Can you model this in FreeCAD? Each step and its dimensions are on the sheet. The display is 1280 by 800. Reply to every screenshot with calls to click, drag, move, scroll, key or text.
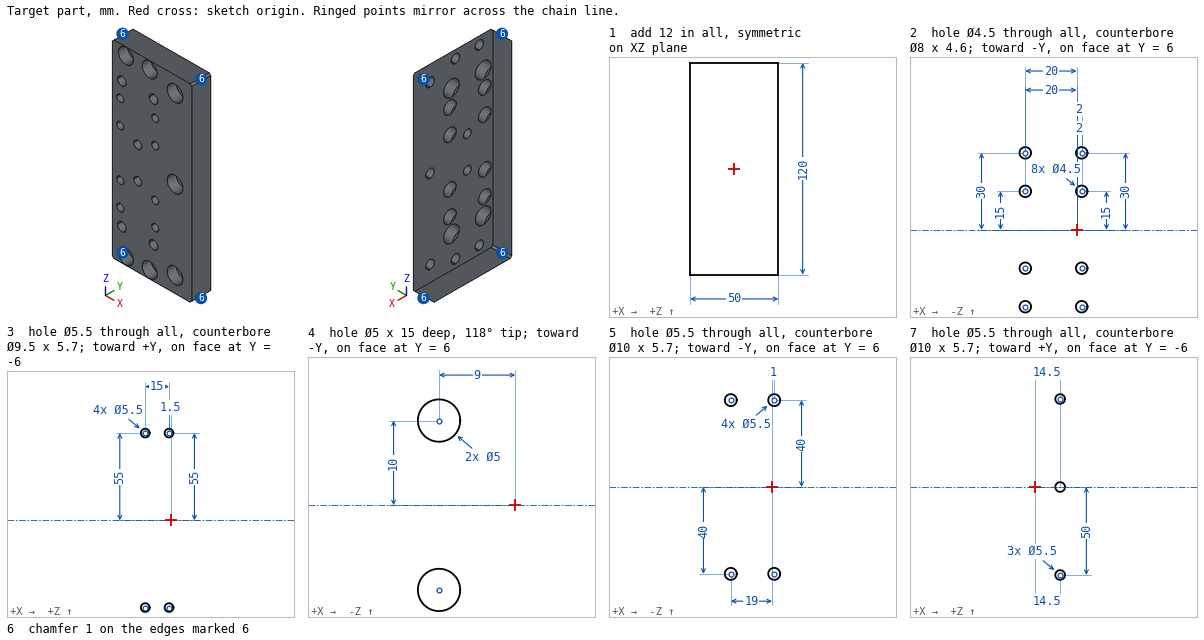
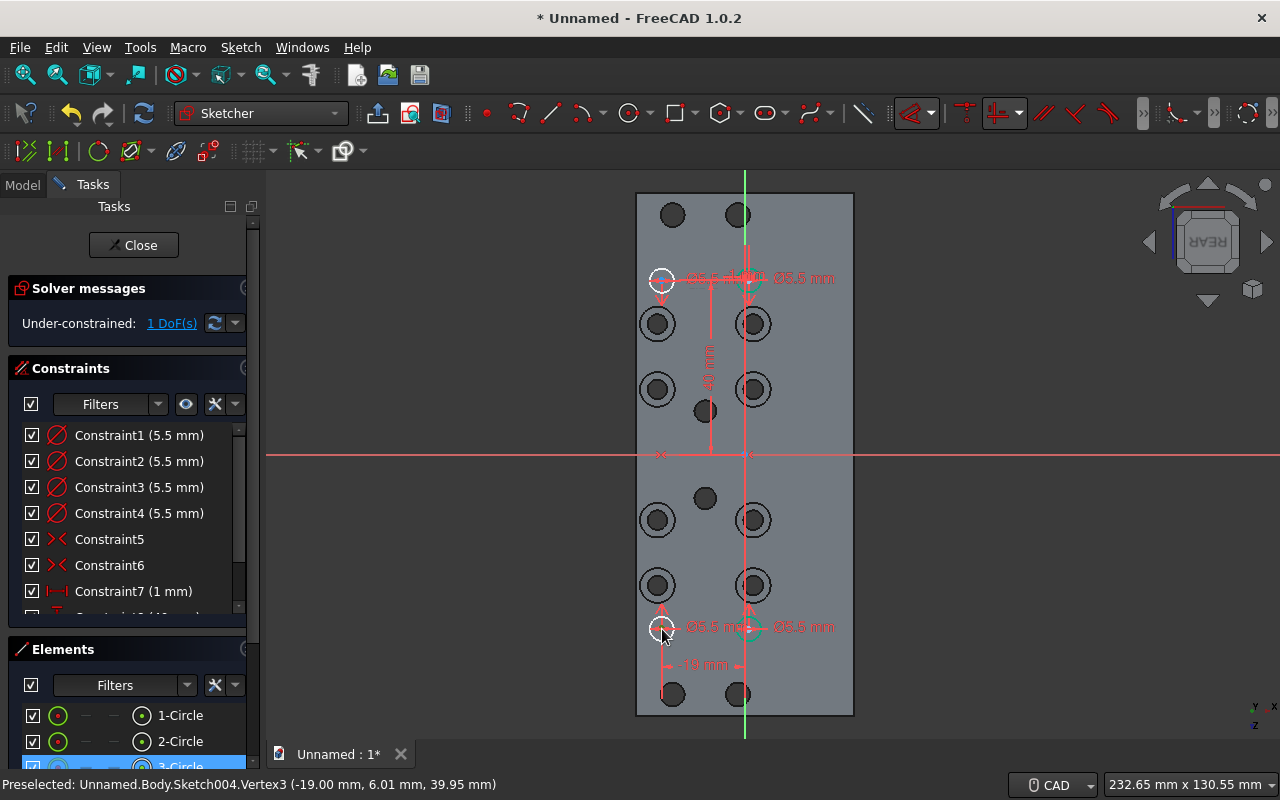
click(934, 114)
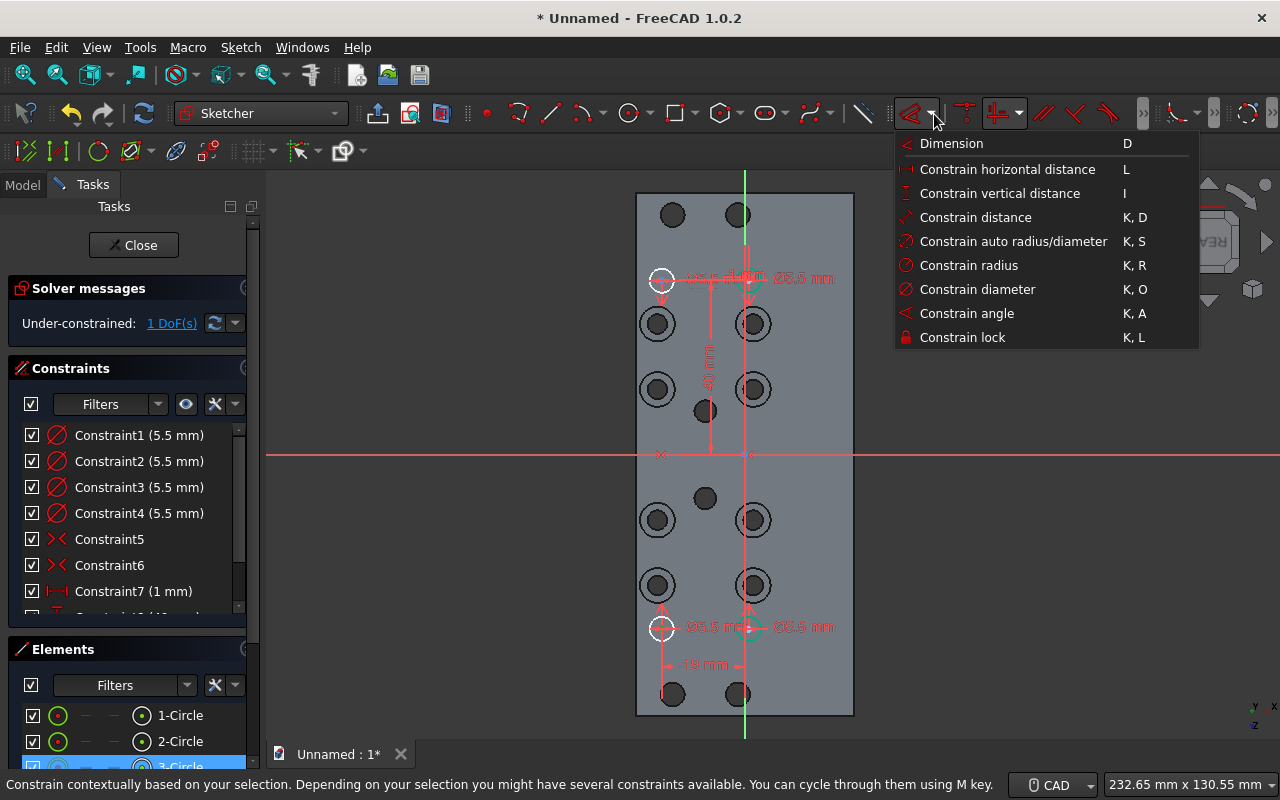
click(1047, 193)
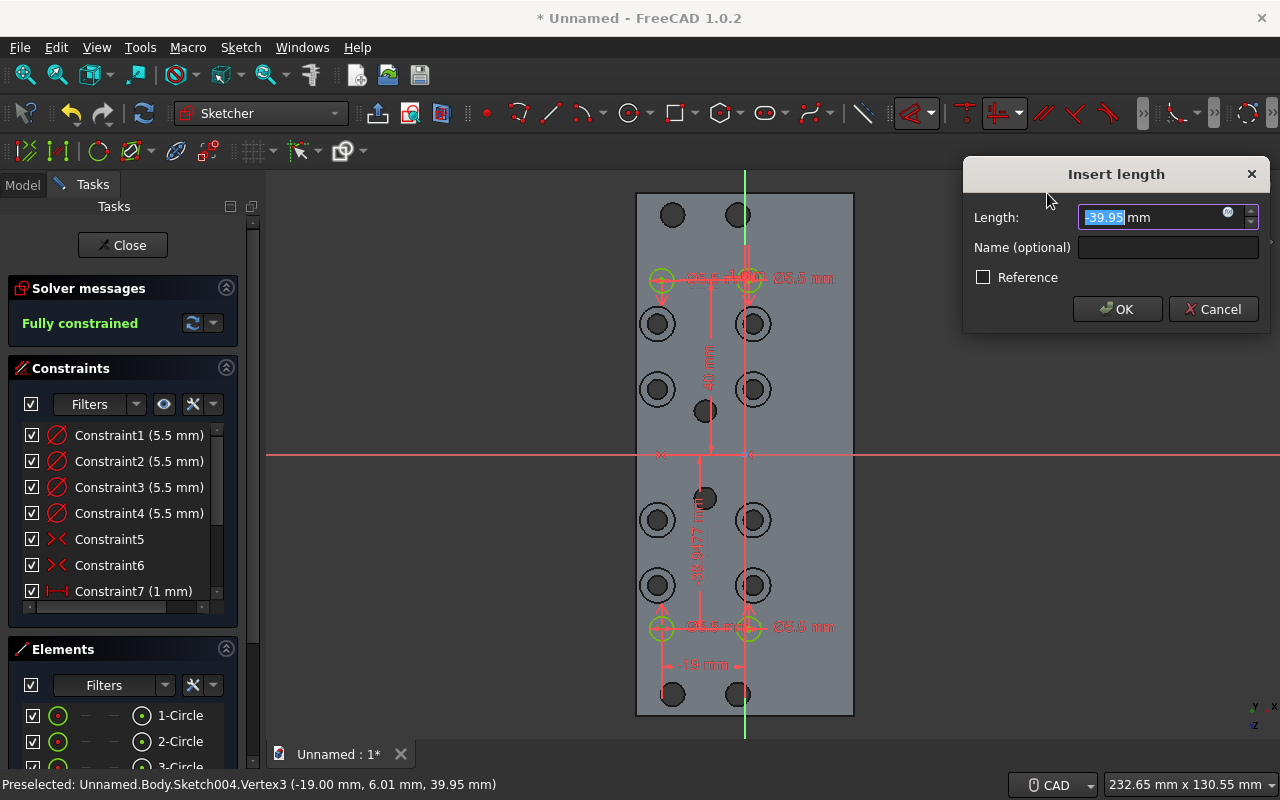
text(-40)
key(Return)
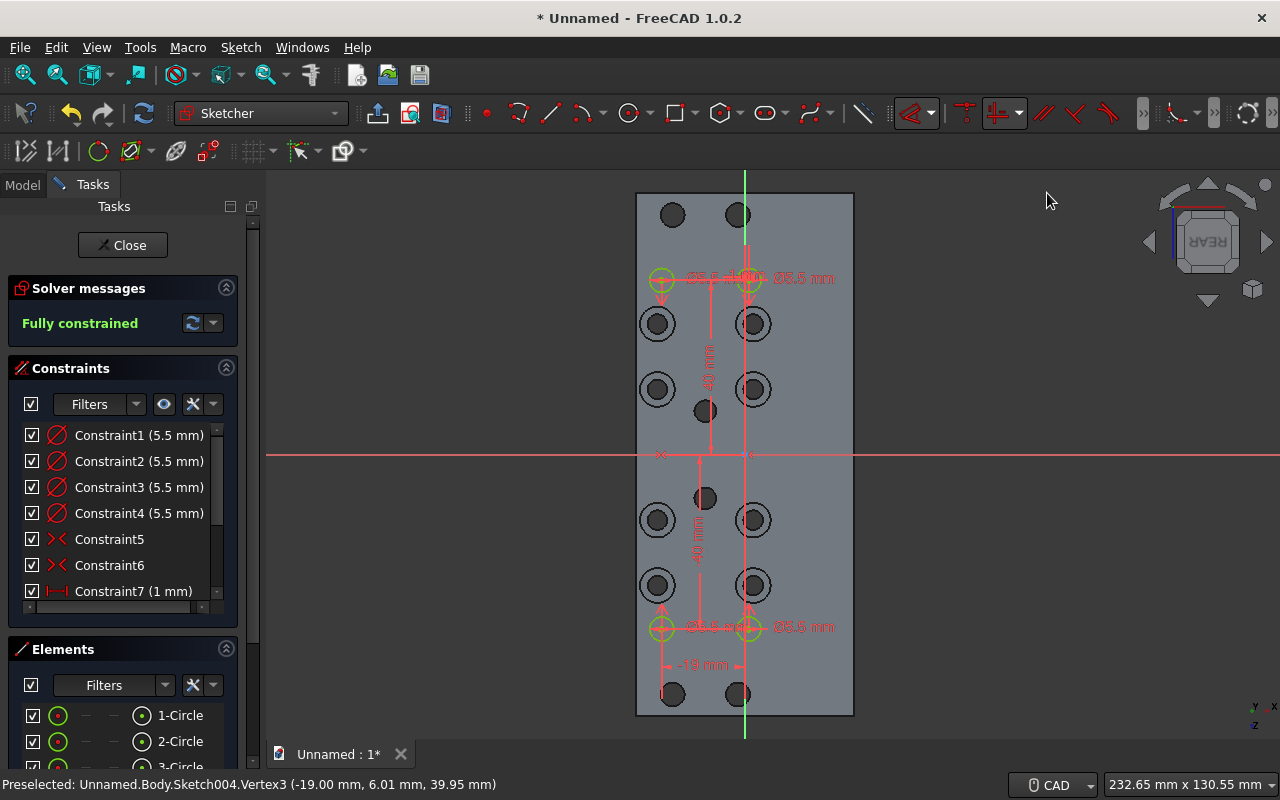
click(123, 245)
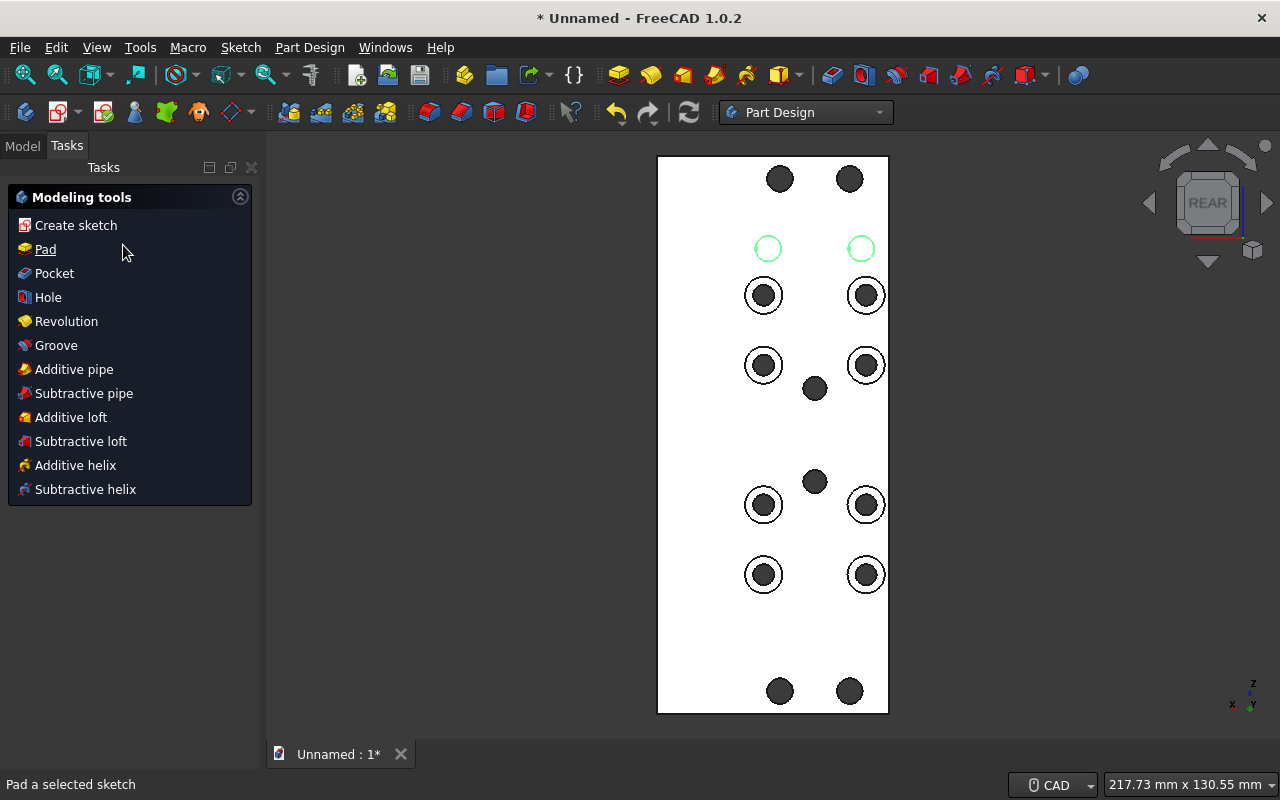
click(866, 76)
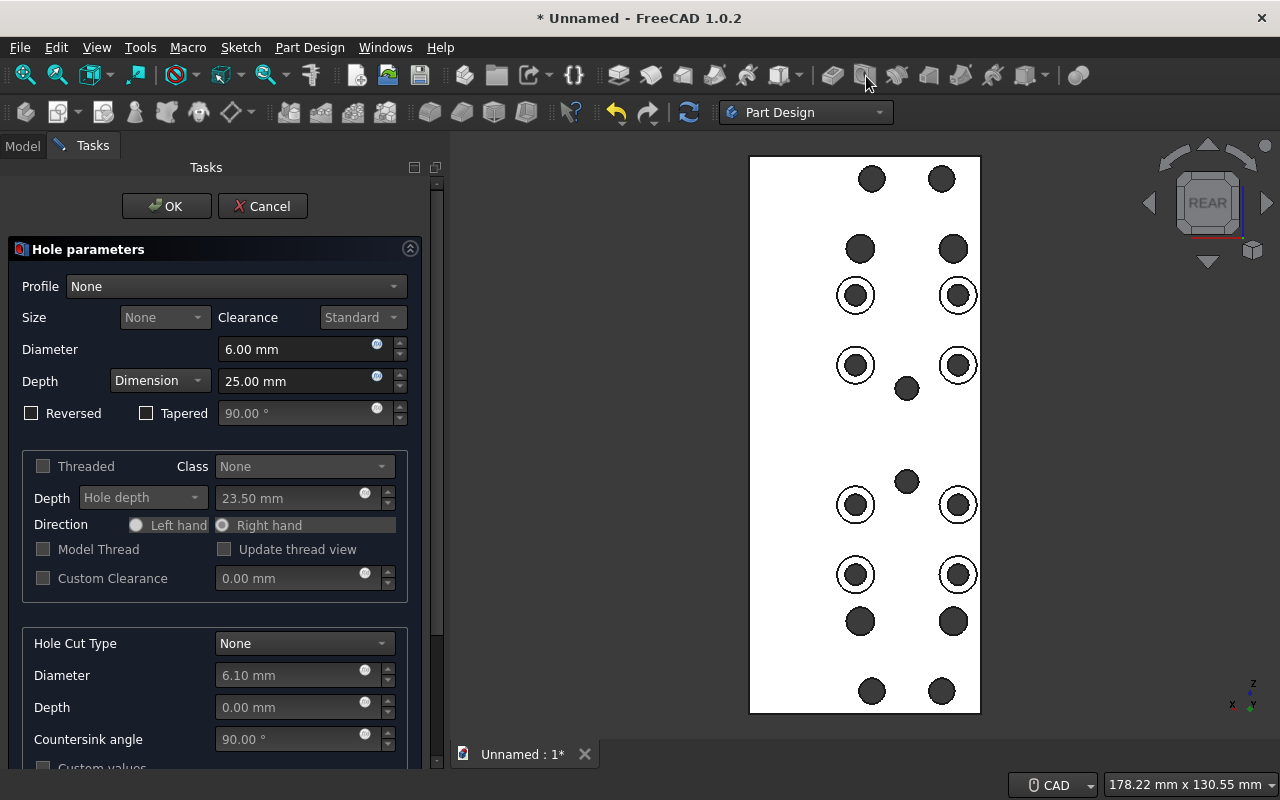
triple_click(305, 349)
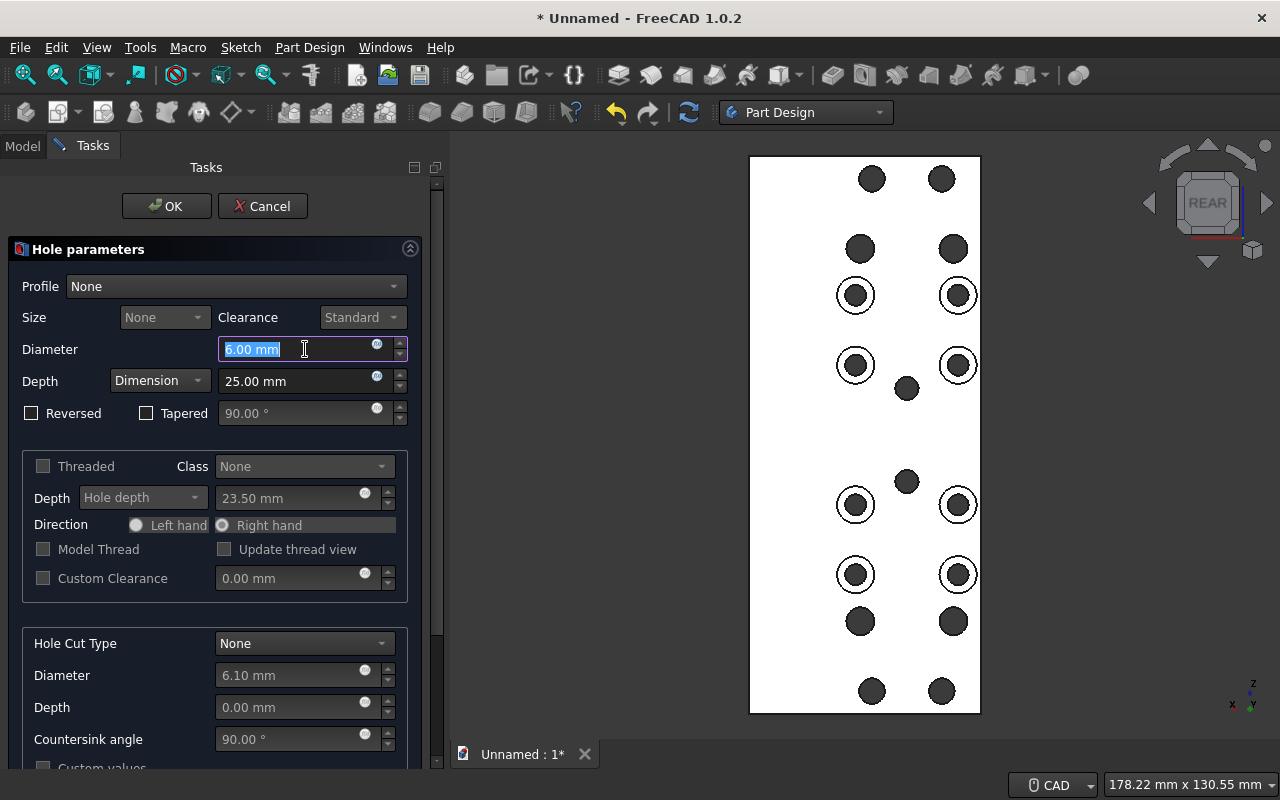
text(5.5)
key(Tab)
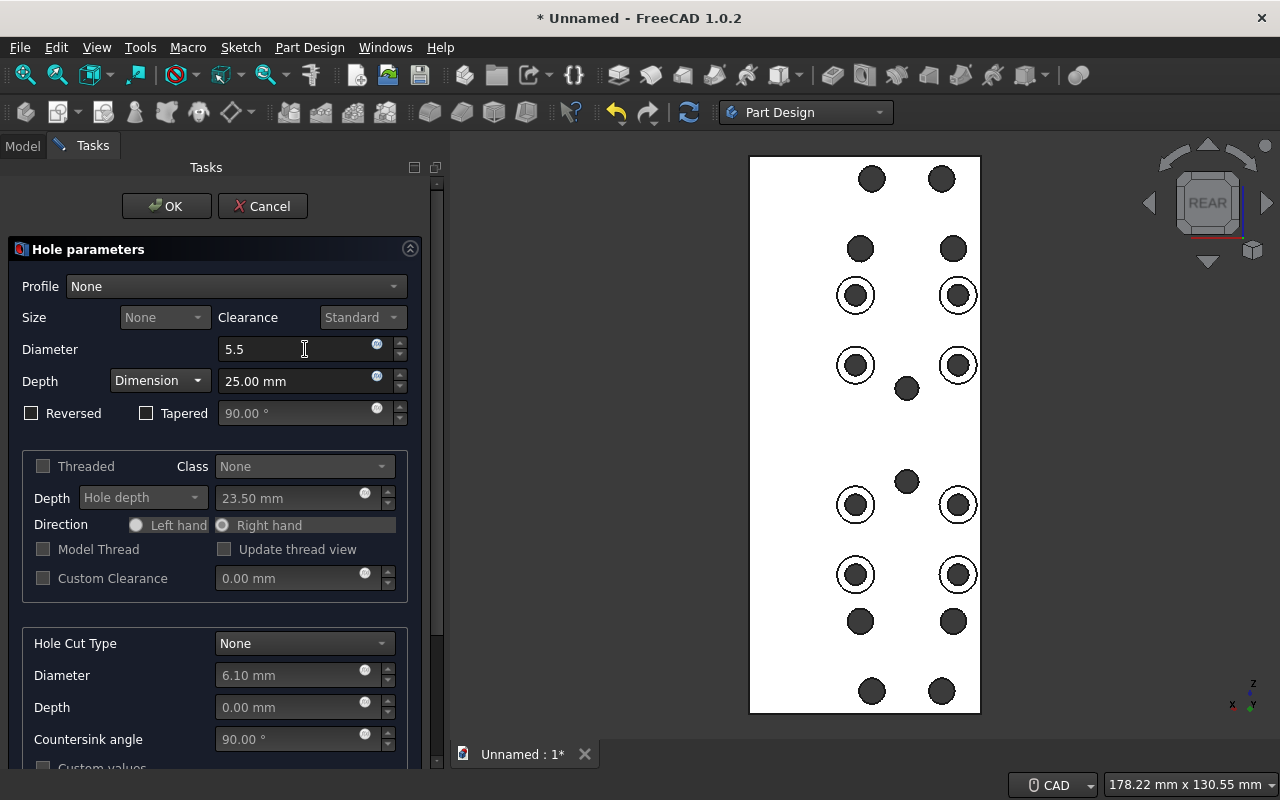
click(161, 380)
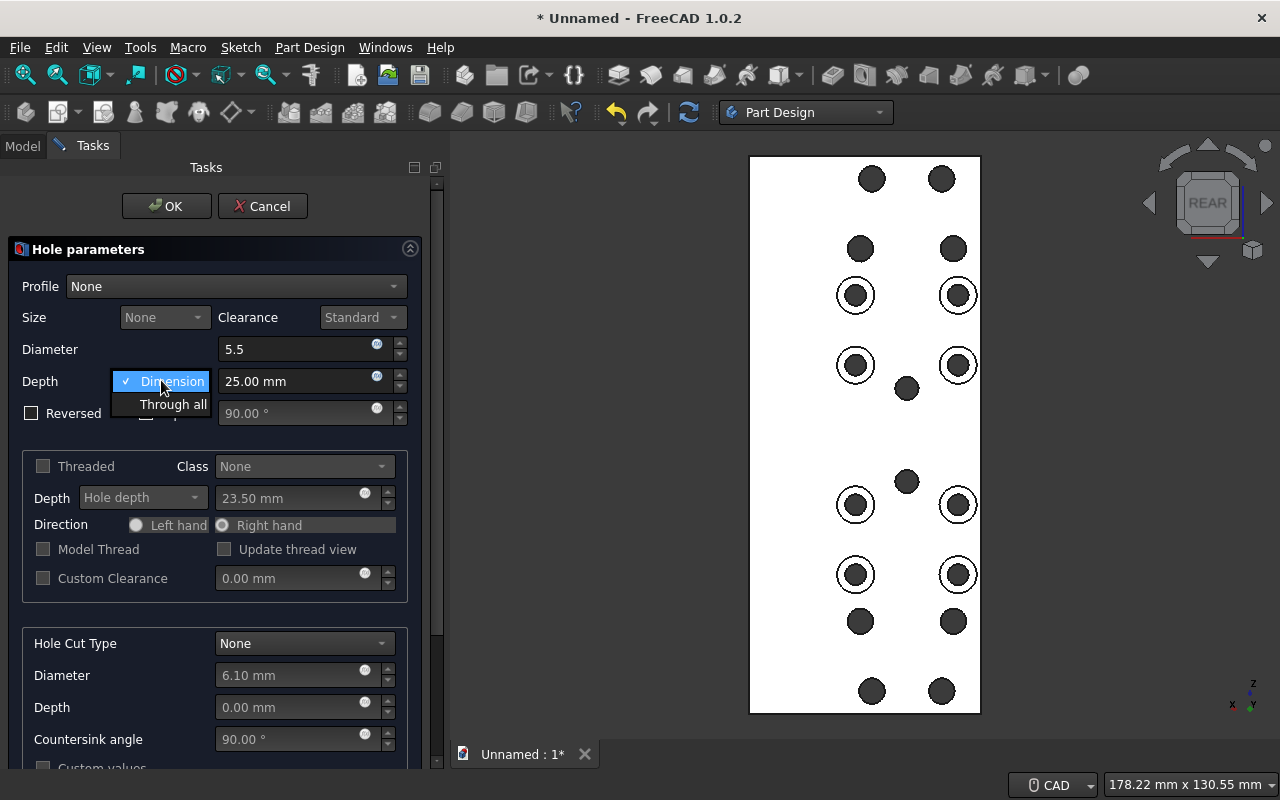
click(160, 404)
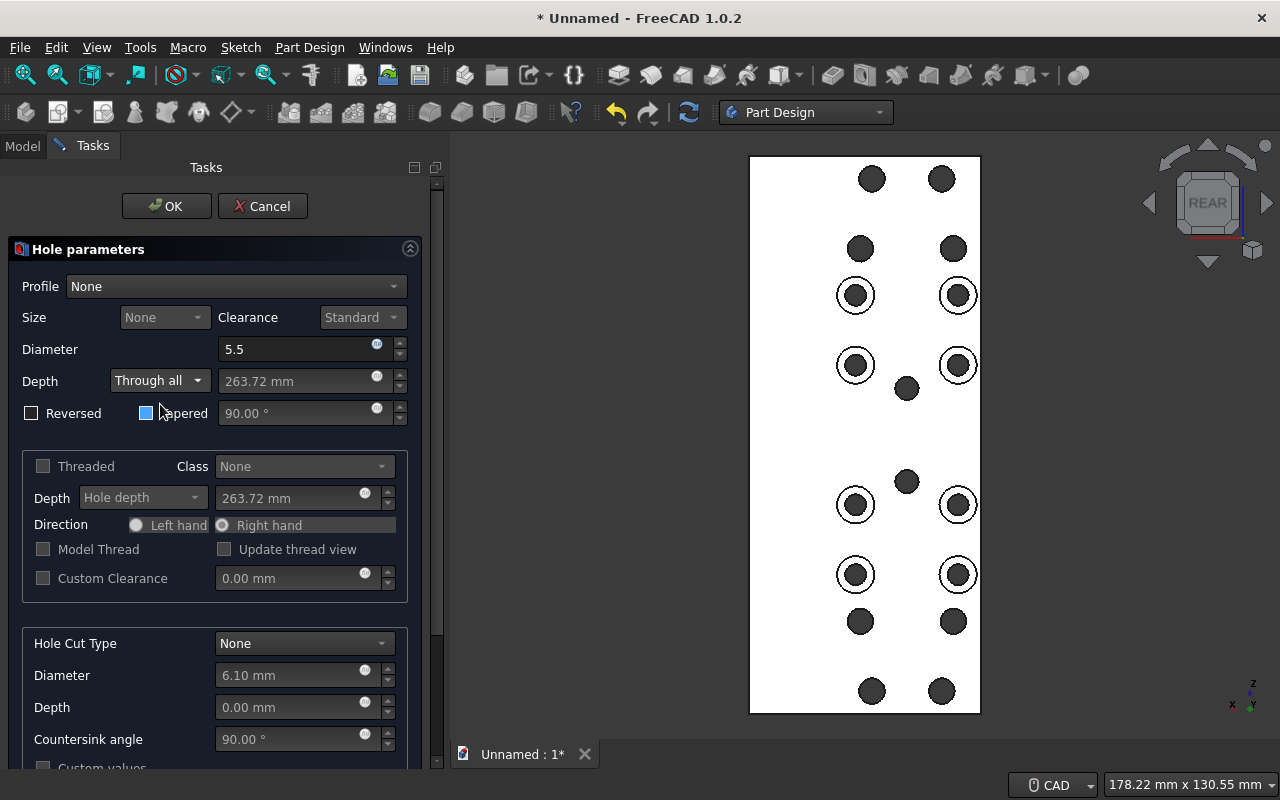
click(306, 644)